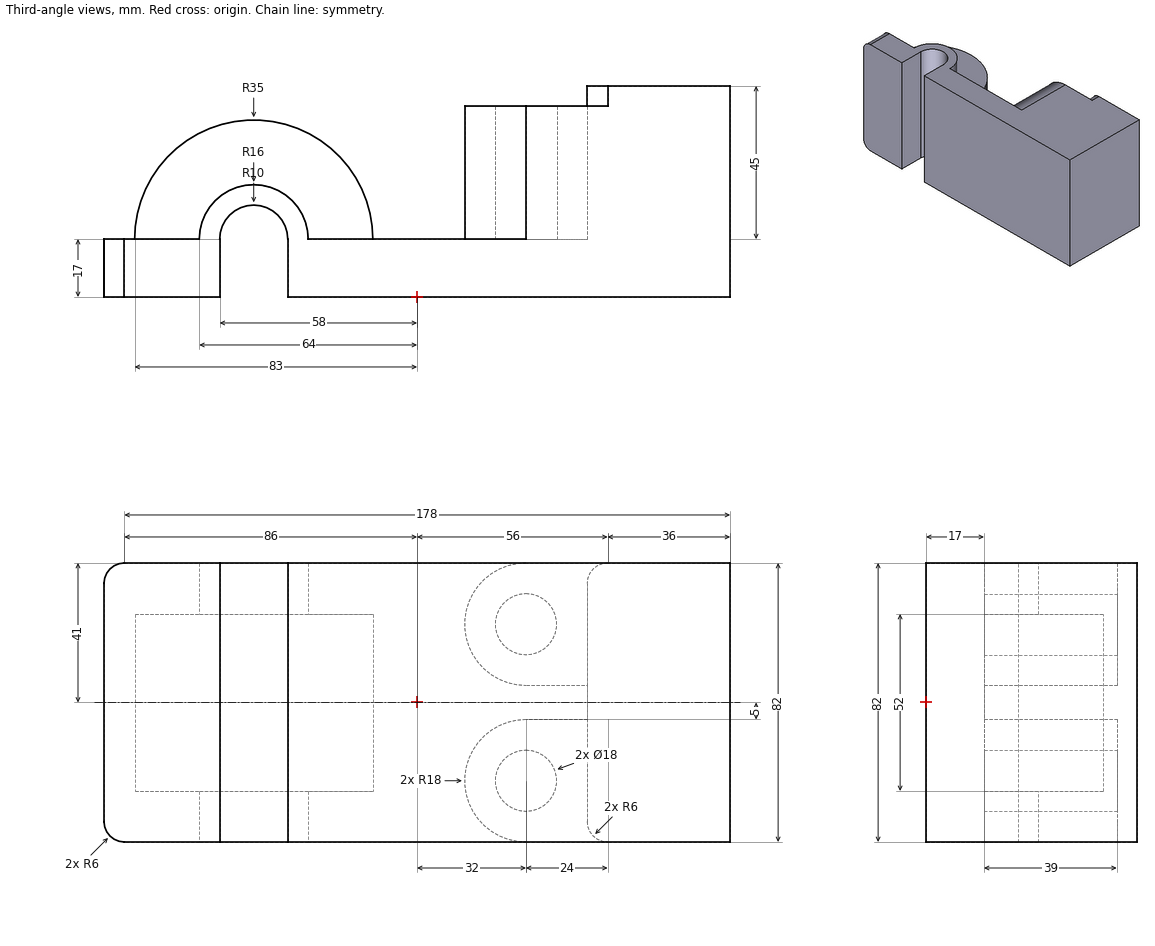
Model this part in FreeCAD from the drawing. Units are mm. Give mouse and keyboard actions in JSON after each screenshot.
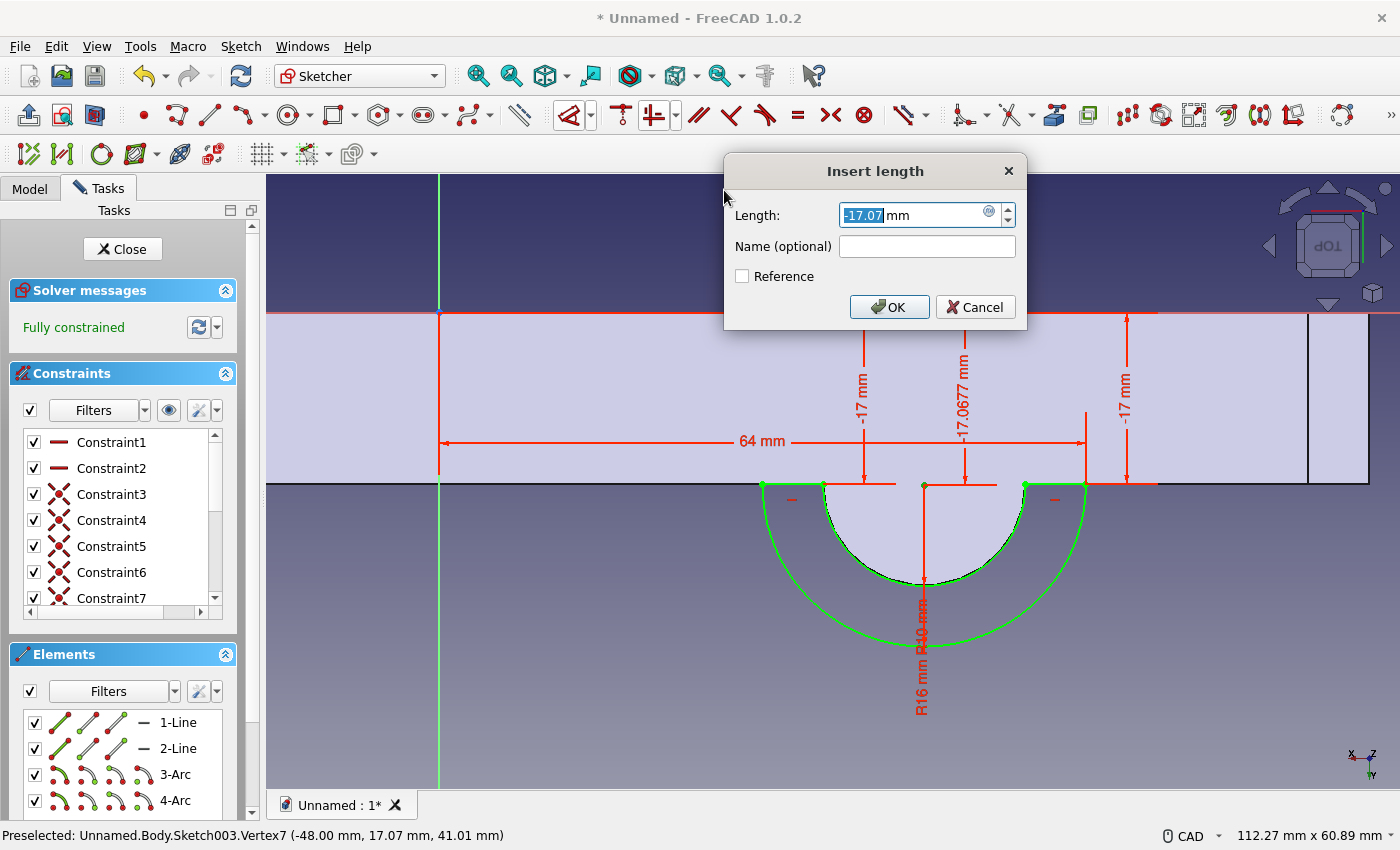
{"action": "type", "text": "-17"}
{"action": "key", "text": "Return"}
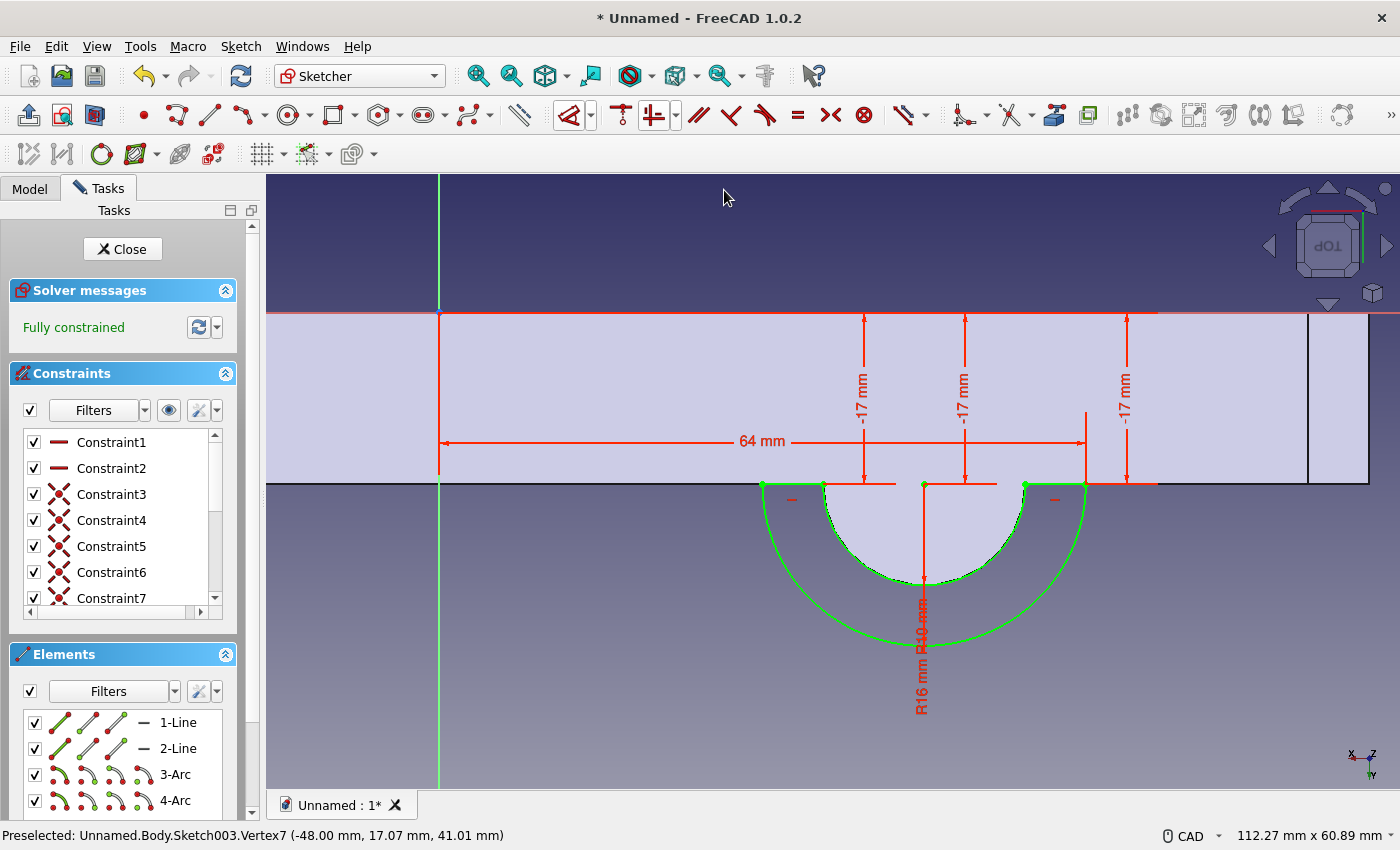
{"action": "left_click", "coordinate": [123, 249]}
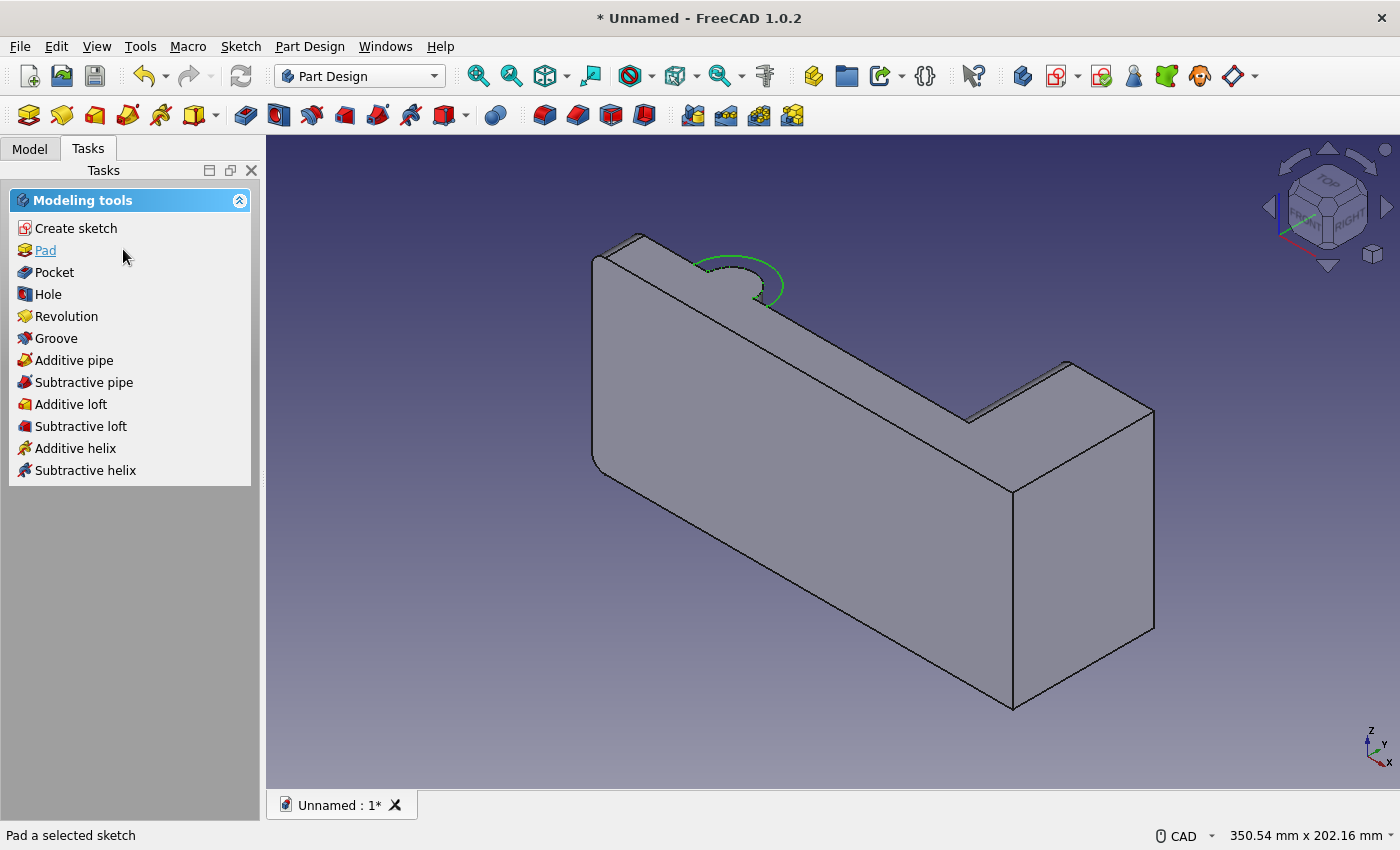
{"action": "left_click", "coordinate": [29, 116]}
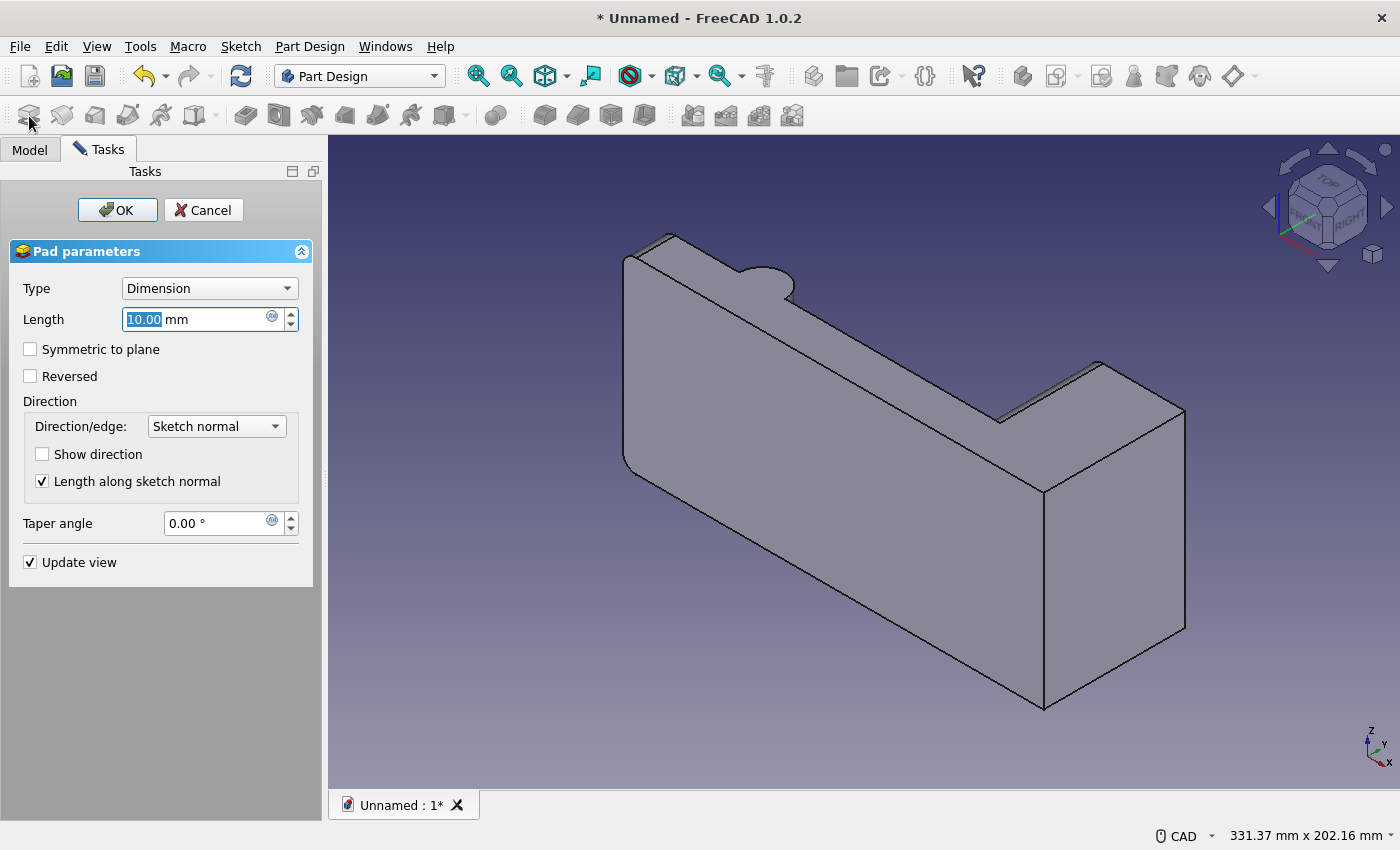
{"action": "type", "text": "82"}
{"action": "key", "text": "Tab"}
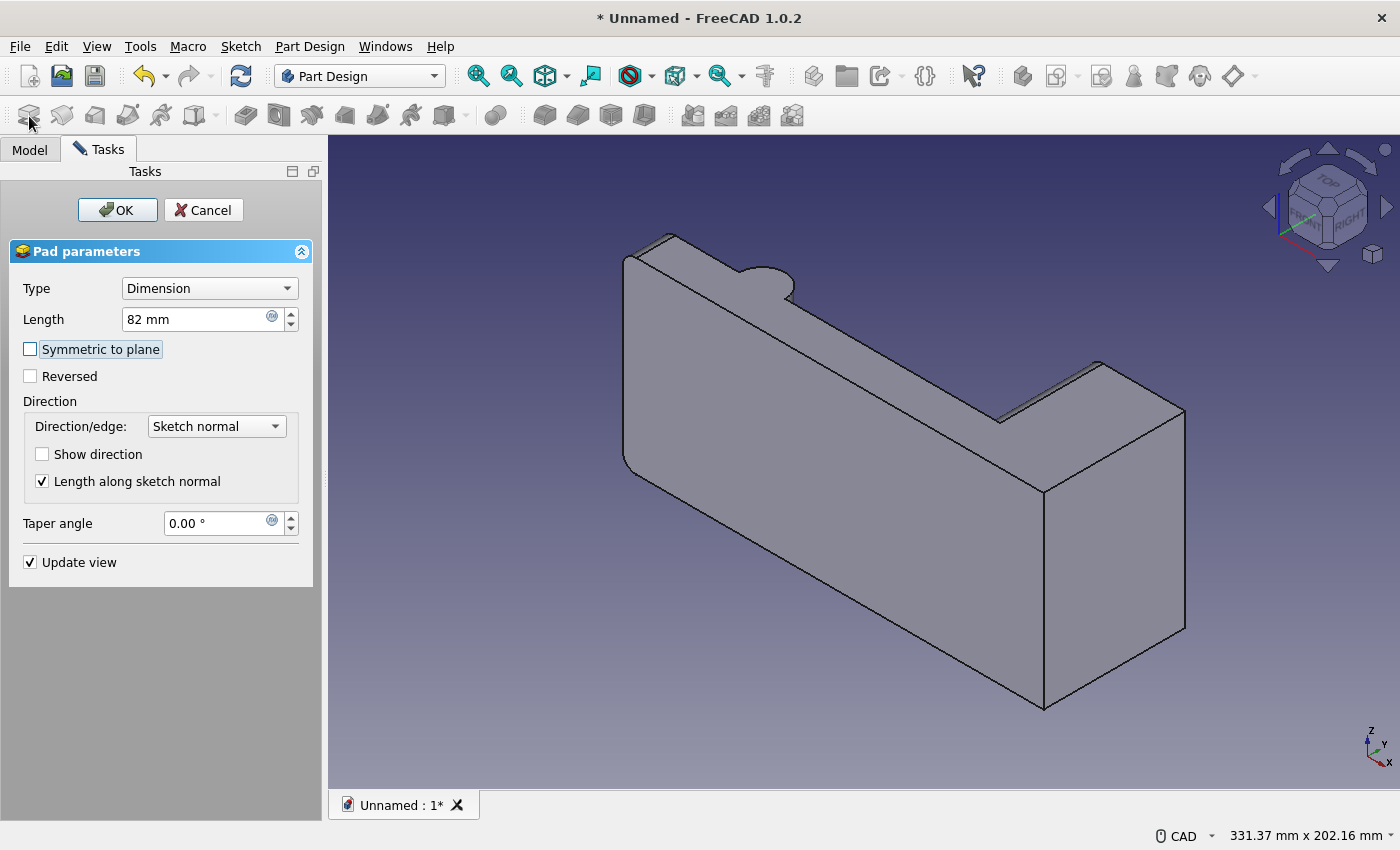
{"action": "left_click", "coordinate": [31, 376]}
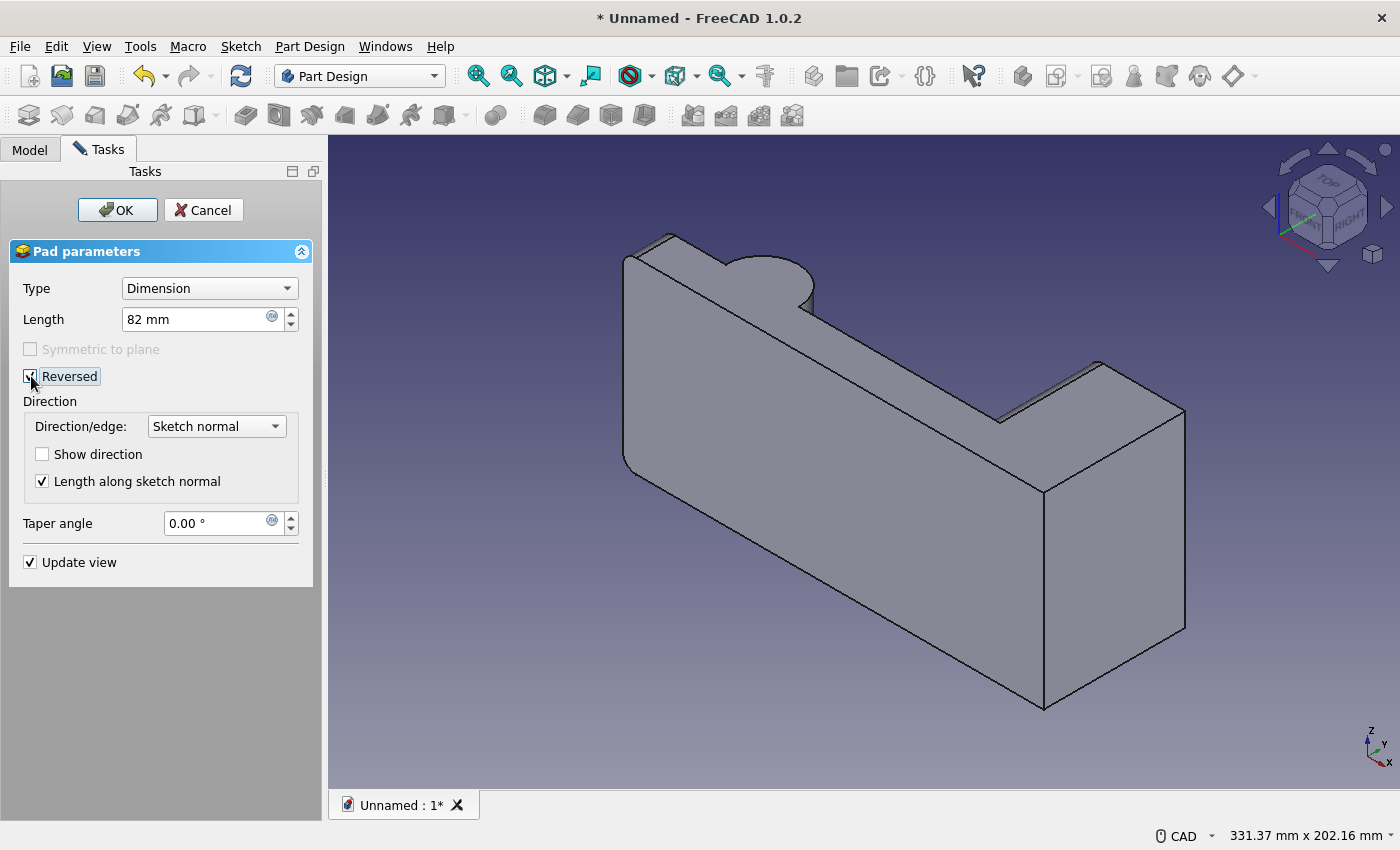
{"action": "left_click", "coordinate": [118, 210]}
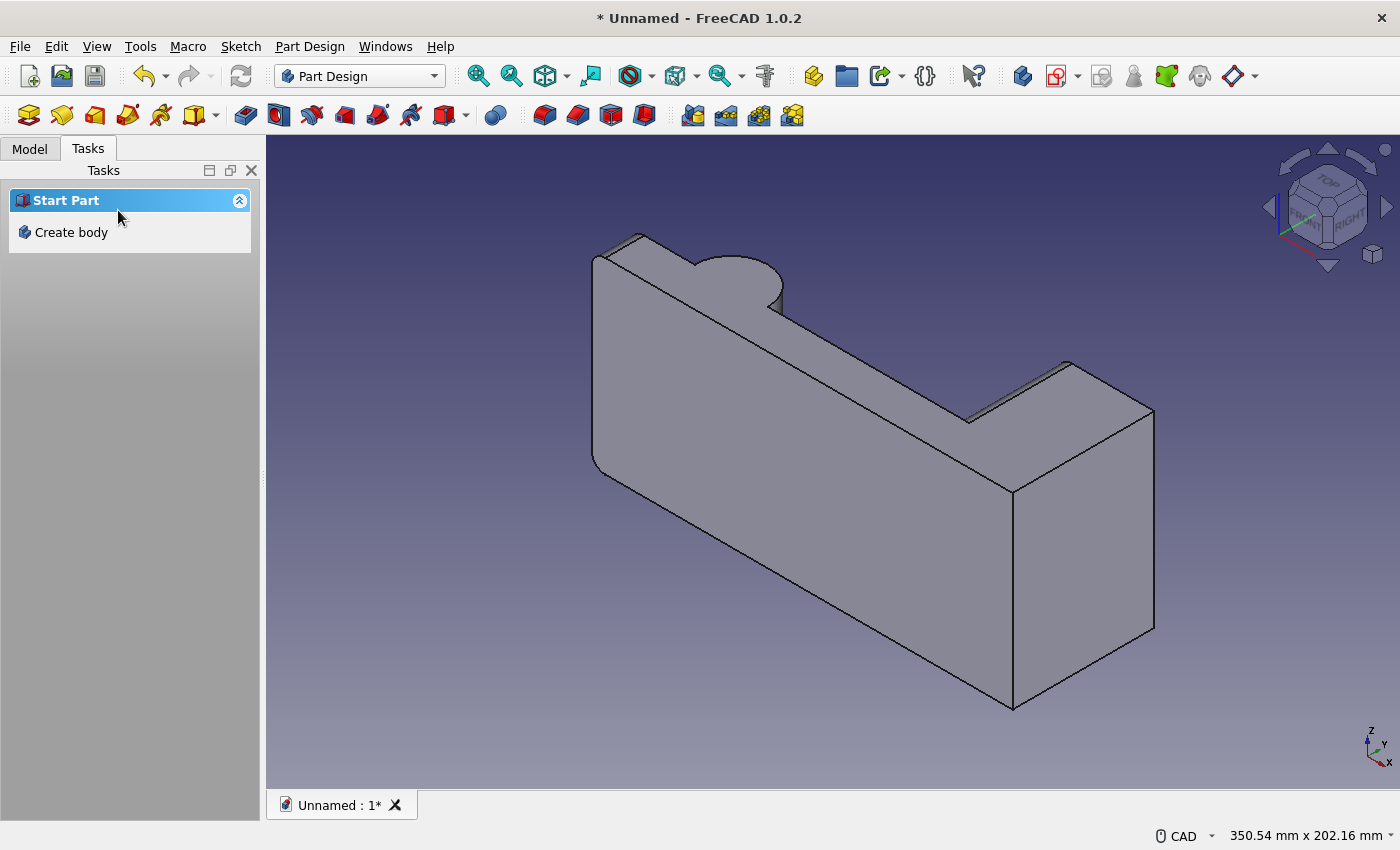
{"action": "left_click", "coordinate": [723, 290]}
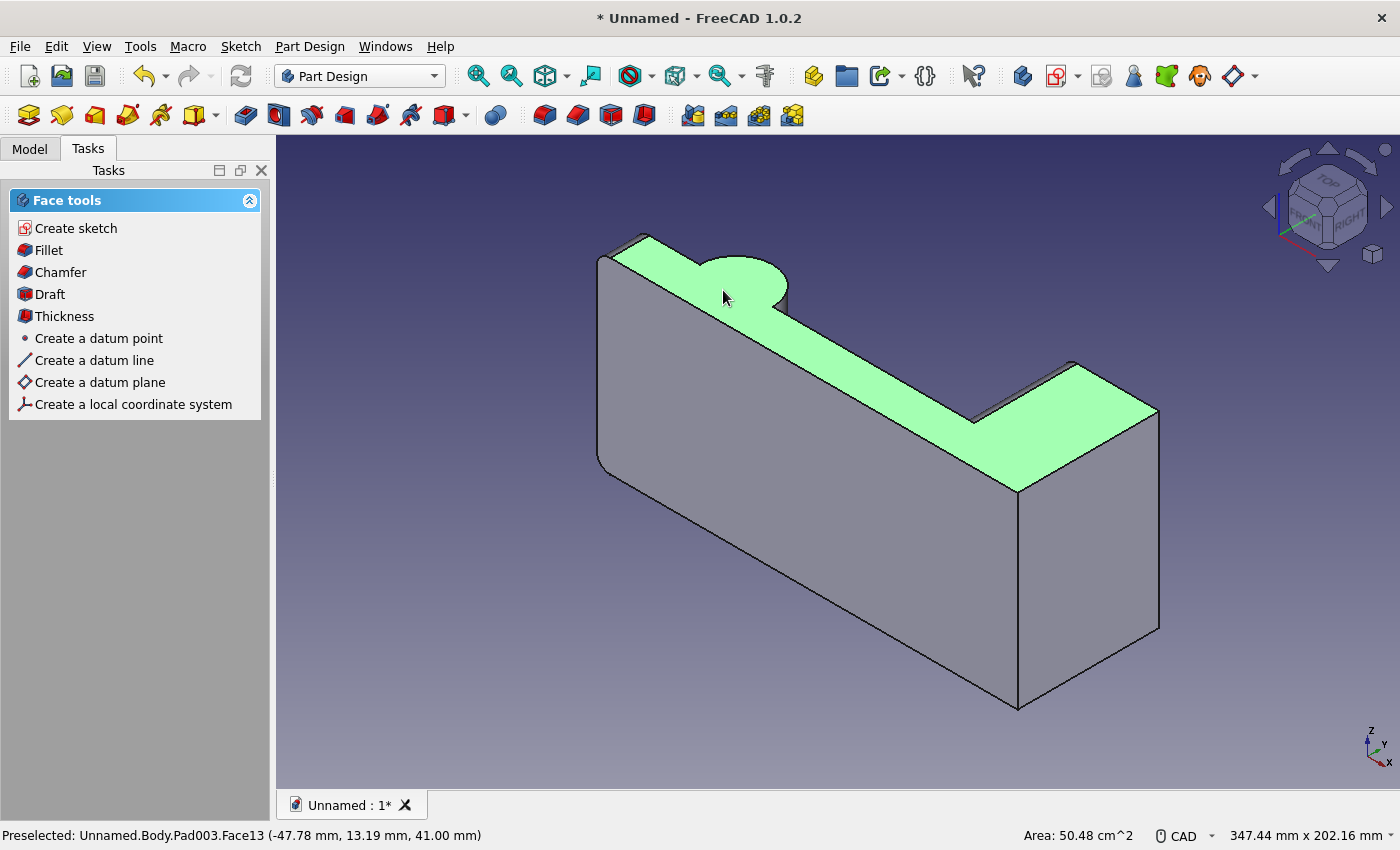
{"action": "left_click", "coordinate": [1056, 76]}